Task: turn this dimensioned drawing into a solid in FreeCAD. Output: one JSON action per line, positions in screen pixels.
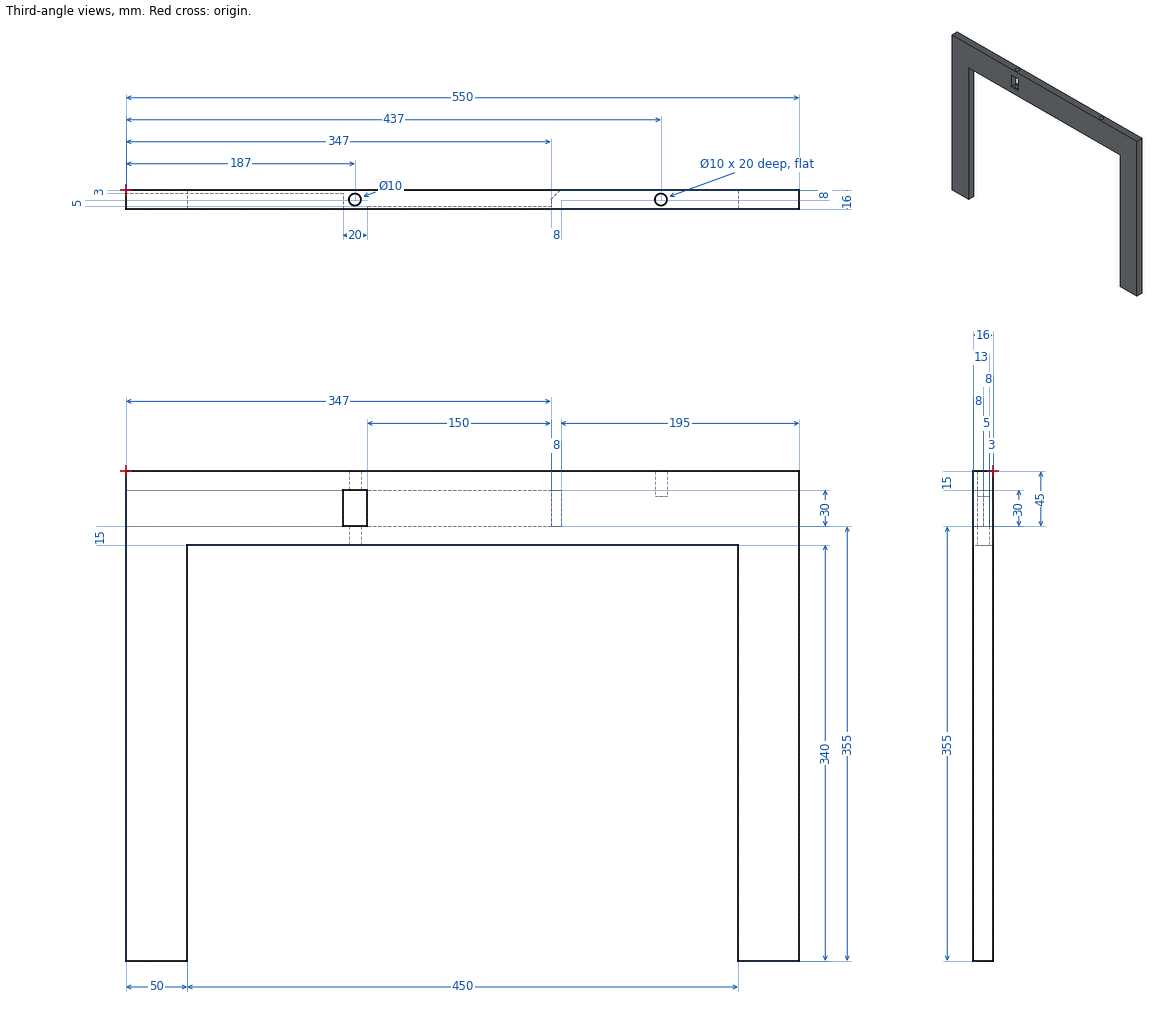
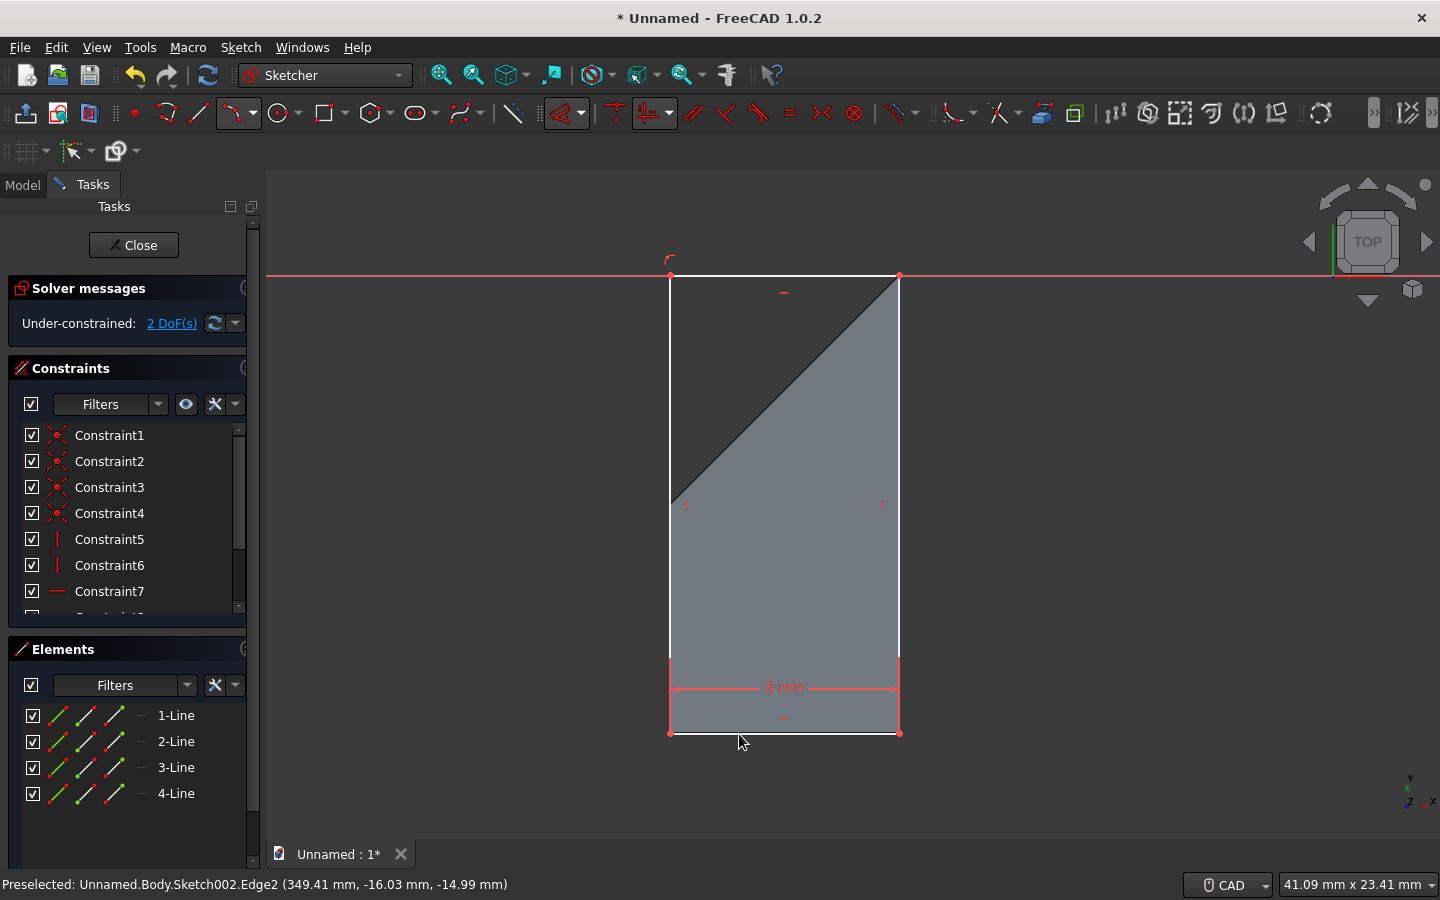
{"action": "left_click", "coordinate": [670, 413]}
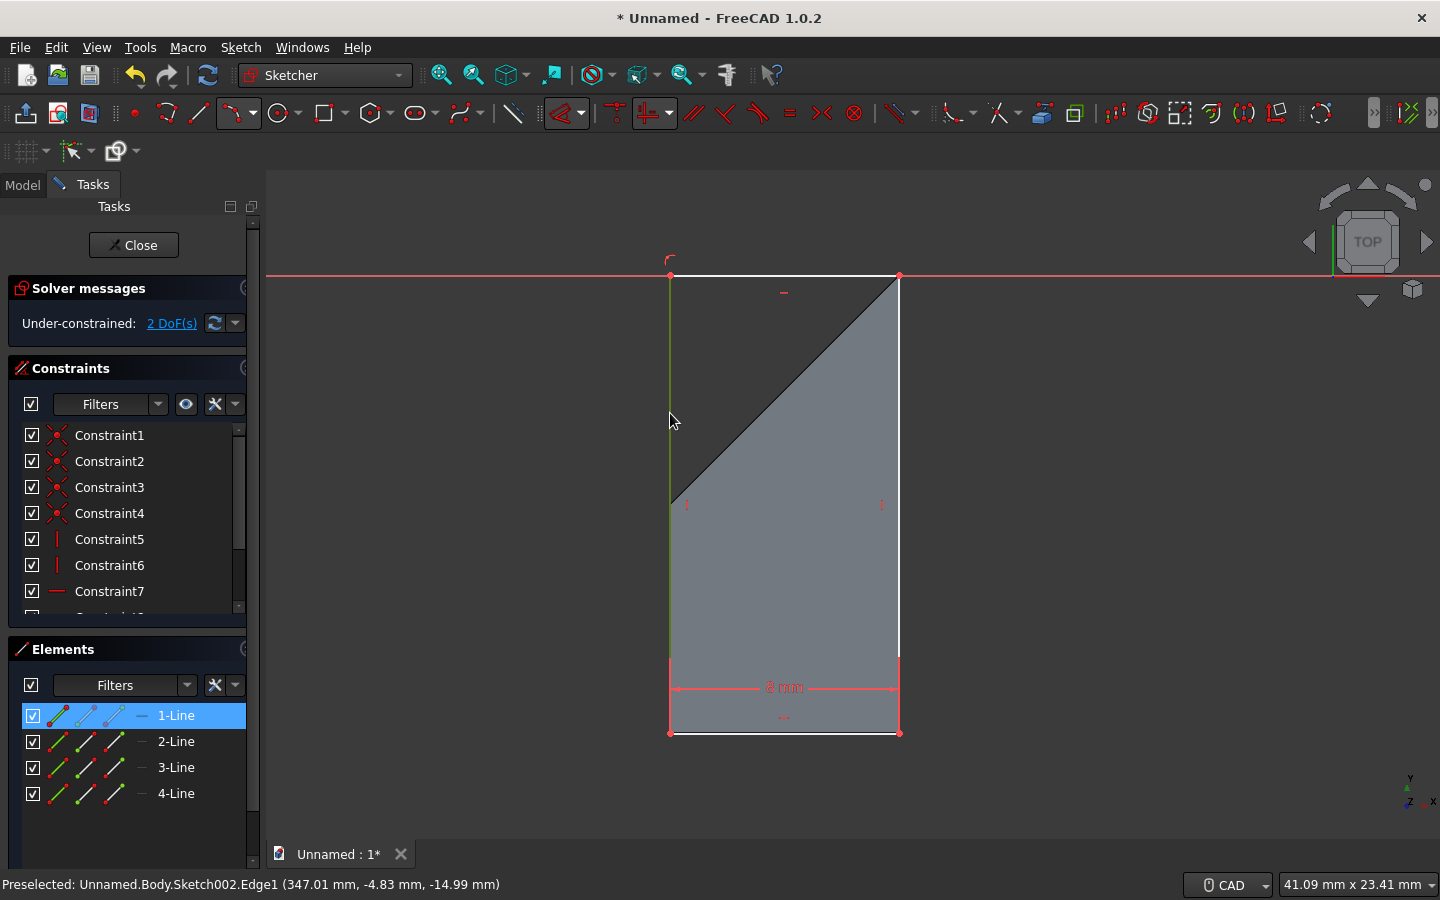
{"action": "key", "text": "i"}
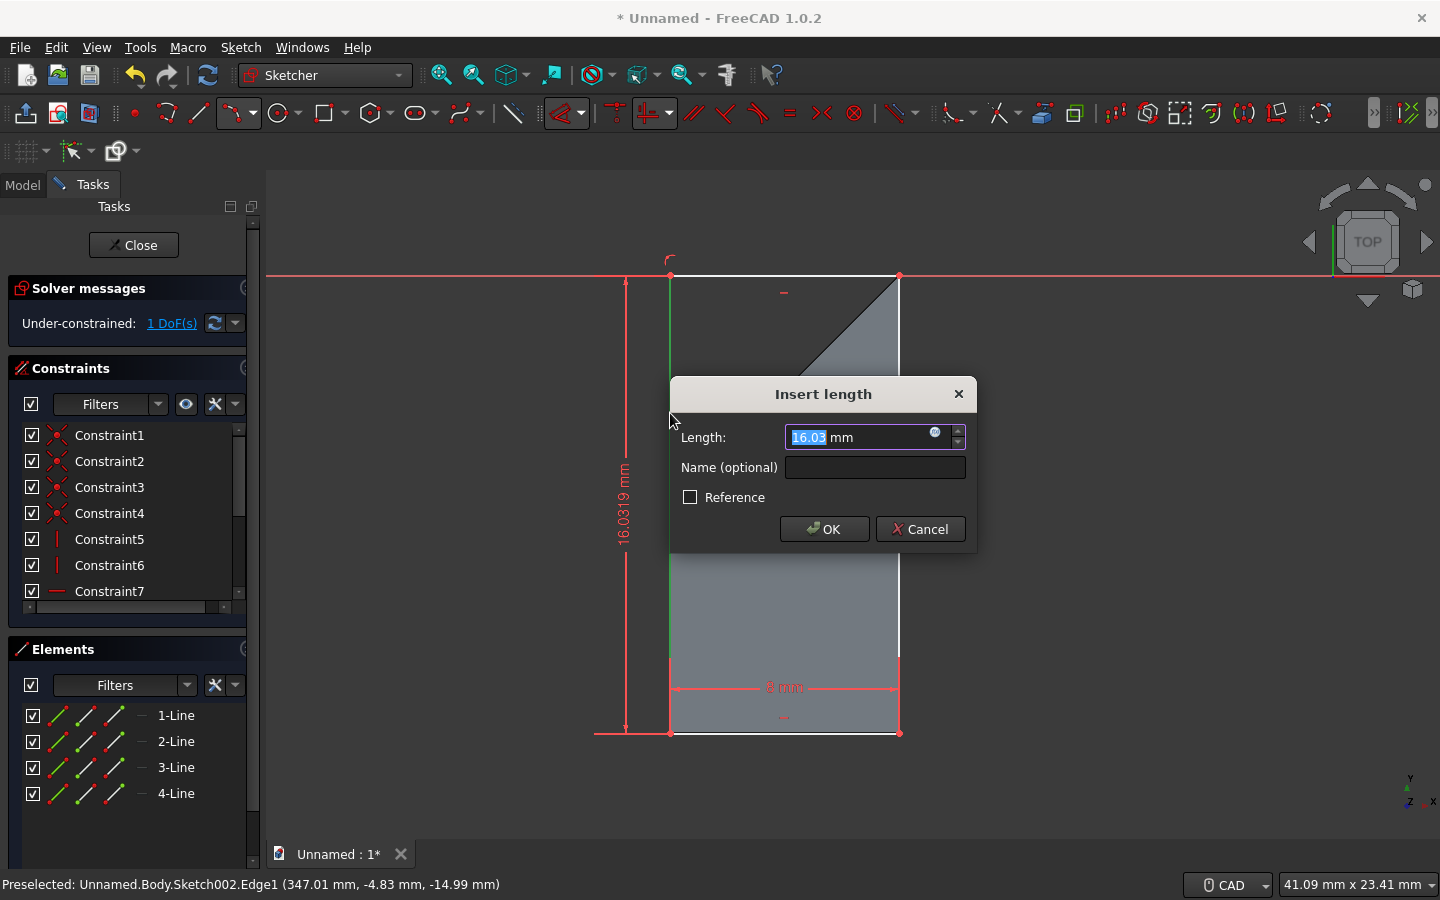
{"action": "type", "text": "16"}
{"action": "key", "text": "Return"}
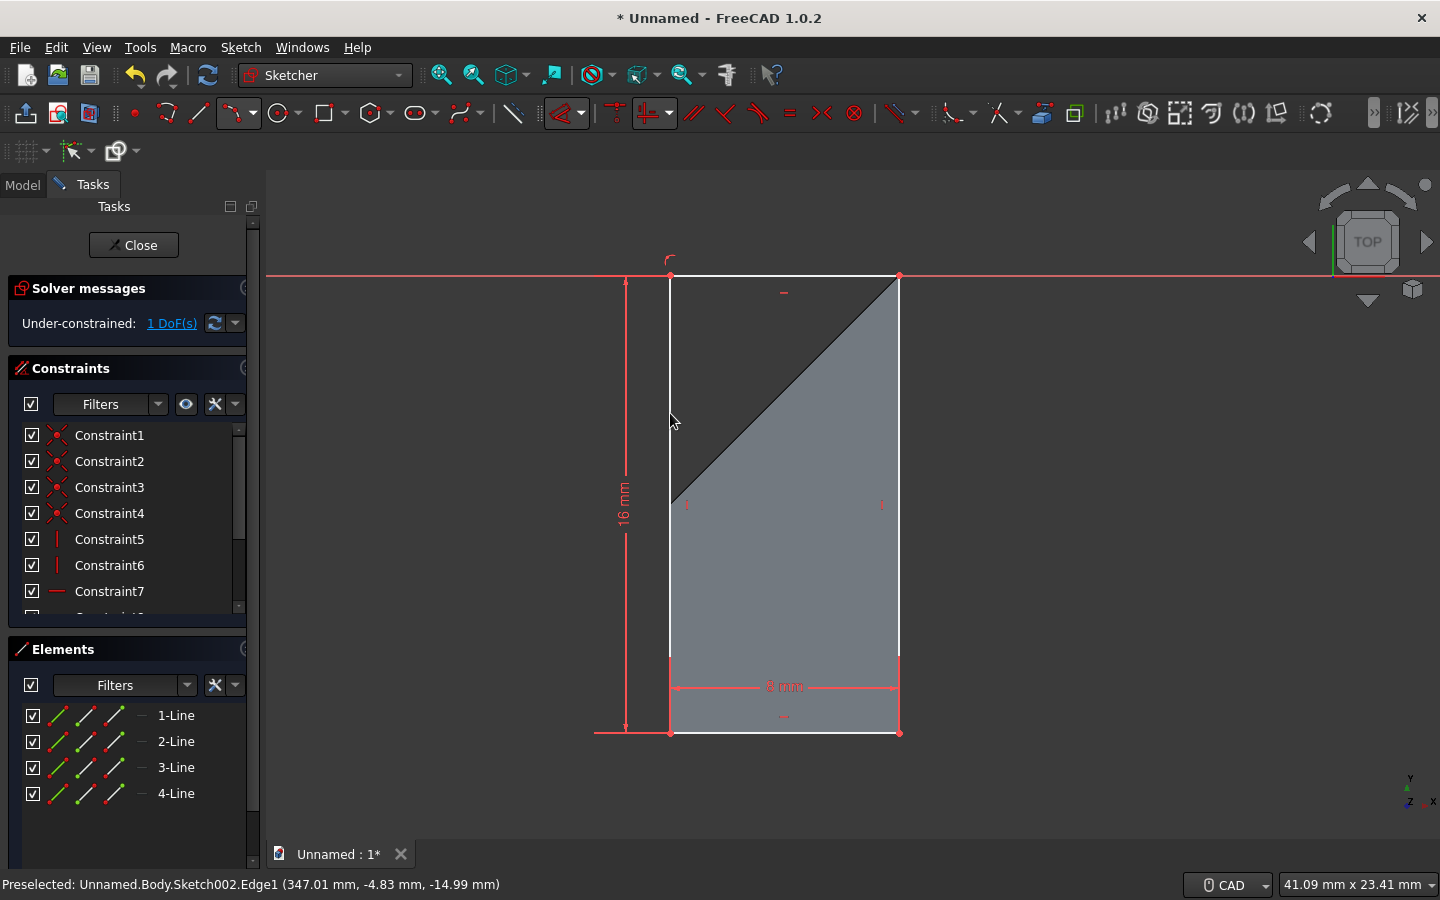
{"action": "left_click", "coordinate": [670, 276]}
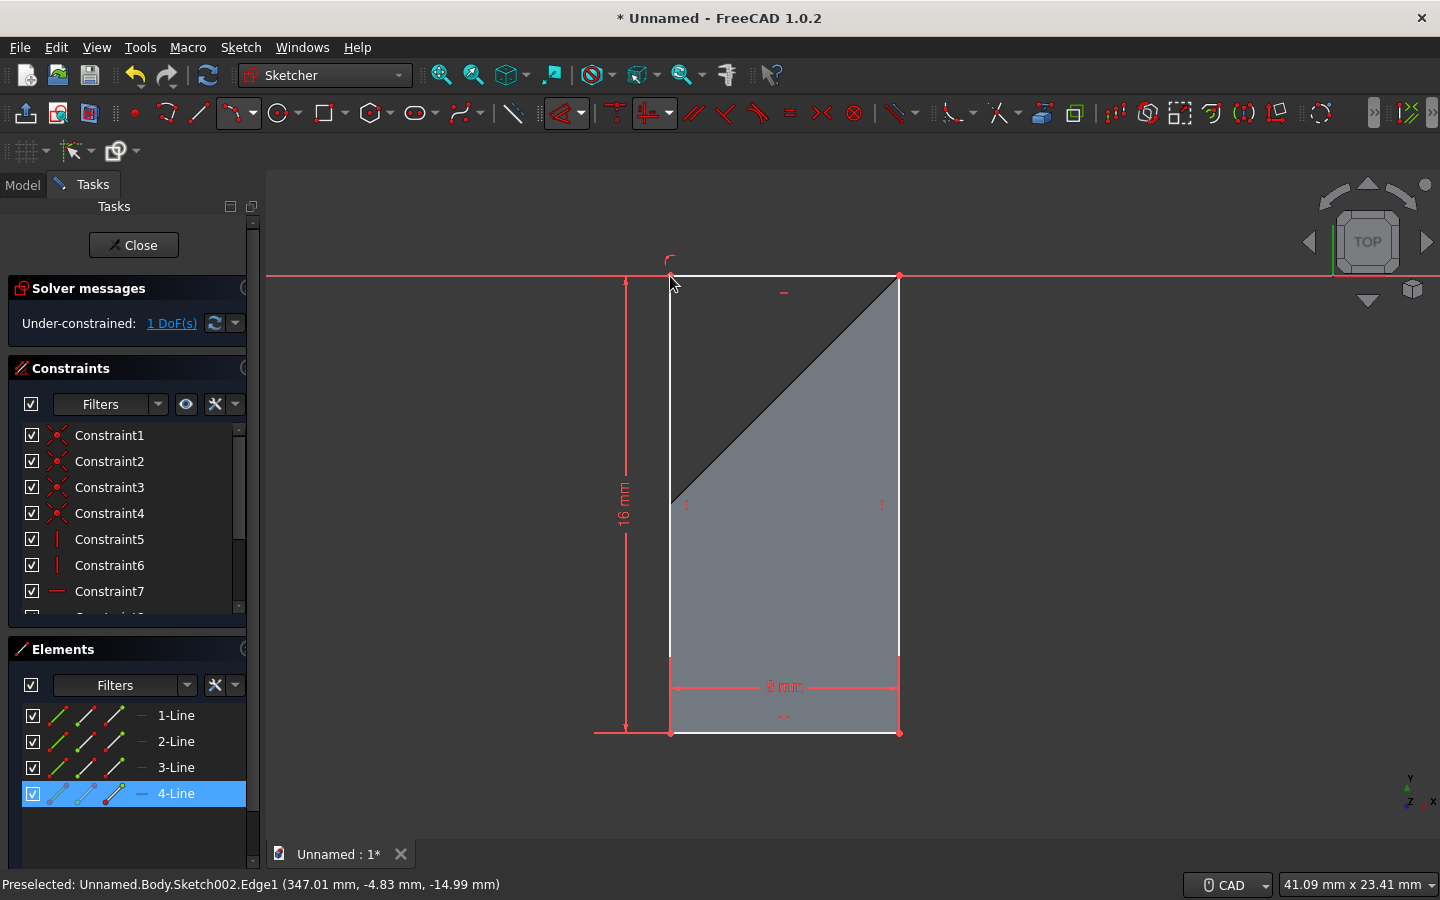
{"action": "left_click", "coordinate": [584, 114]}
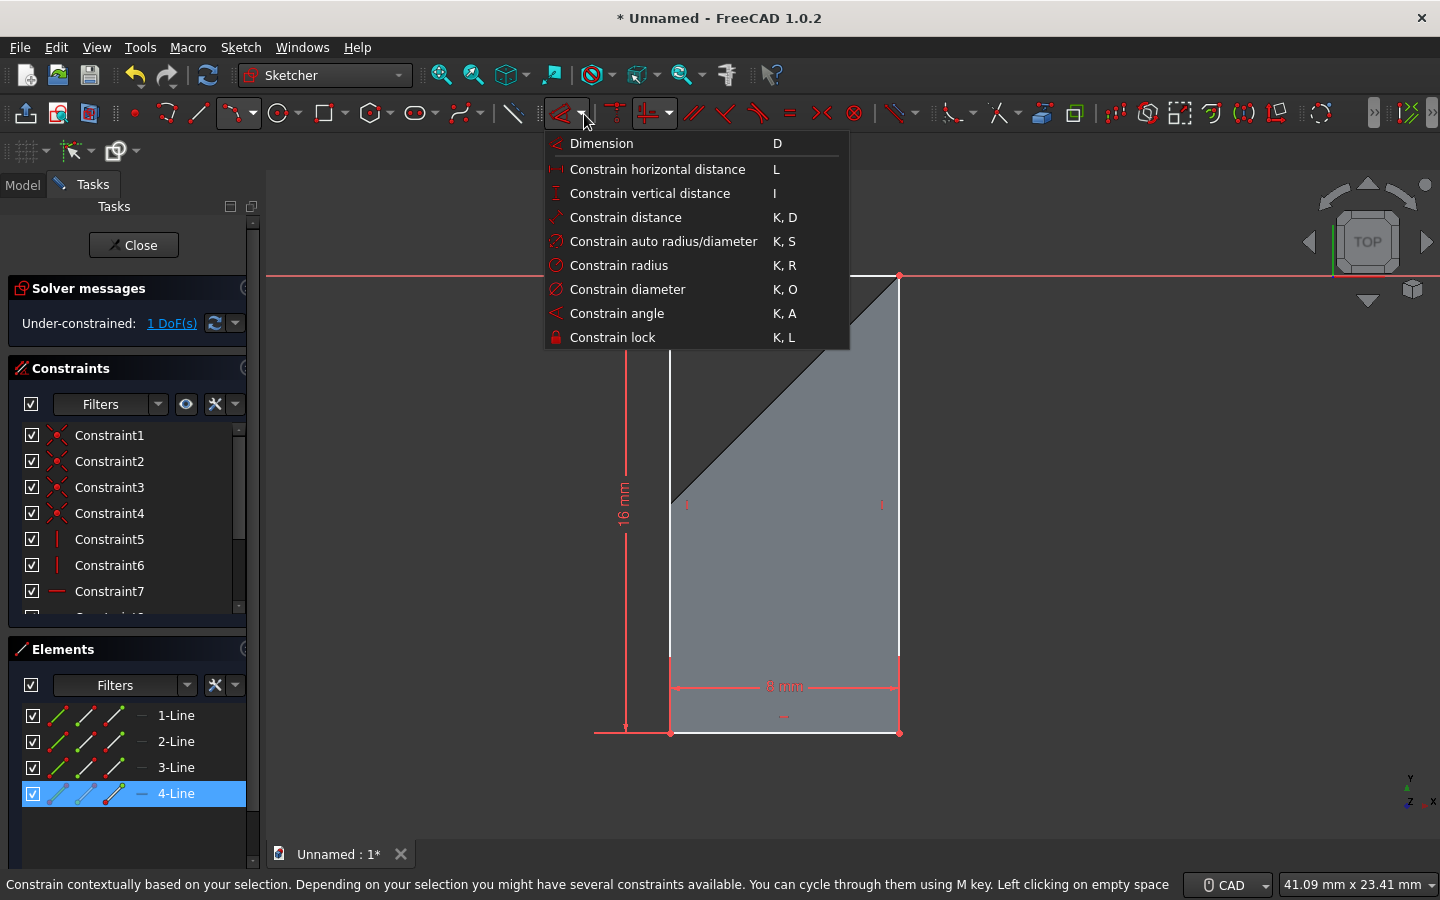
{"action": "left_click", "coordinate": [697, 169]}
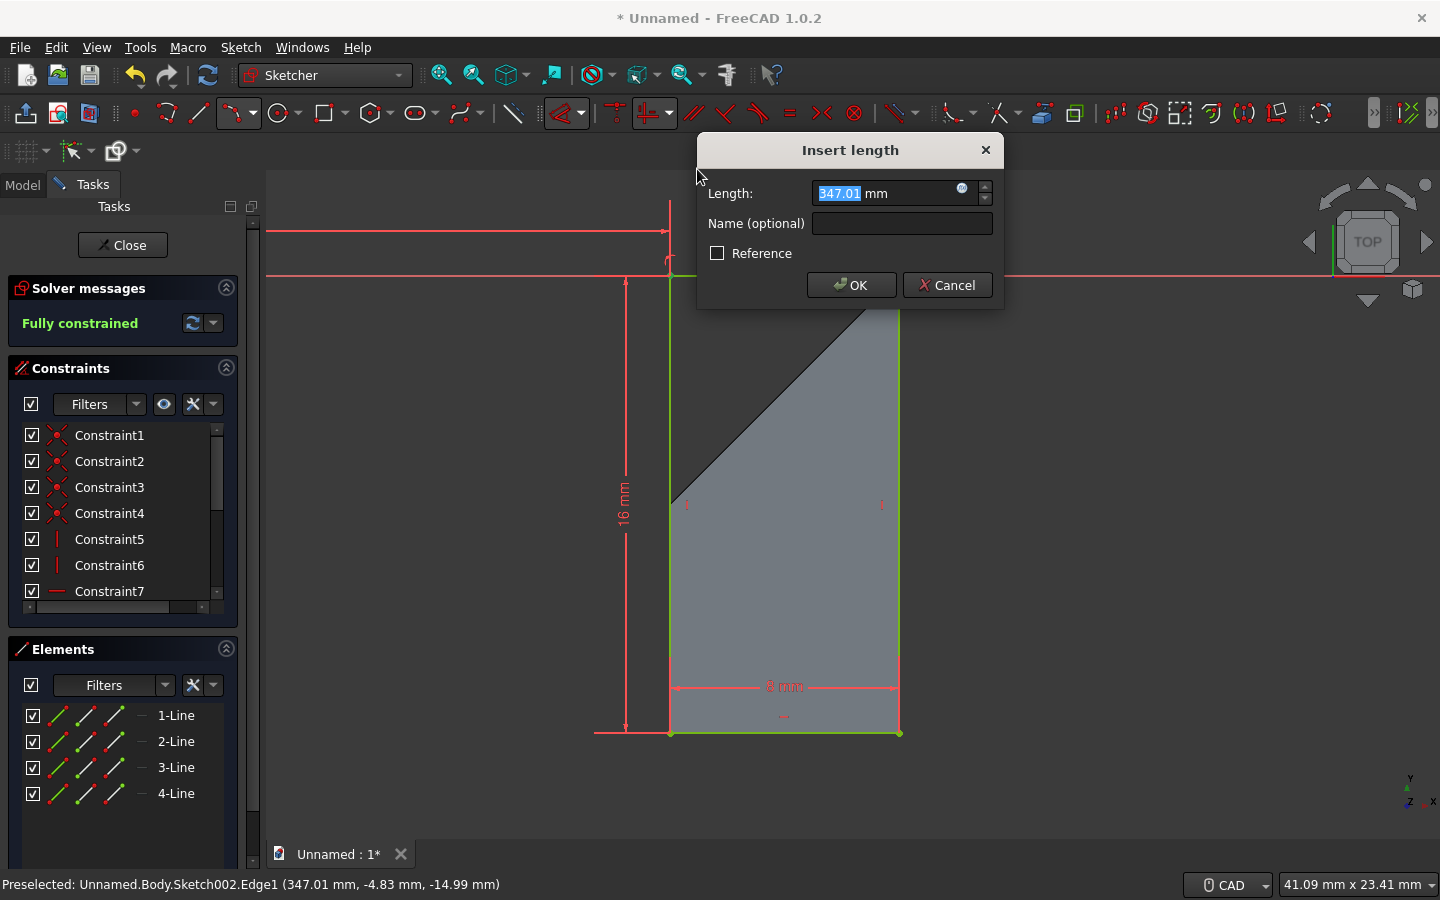
{"action": "type", "text": "347"}
{"action": "key", "text": "Return"}